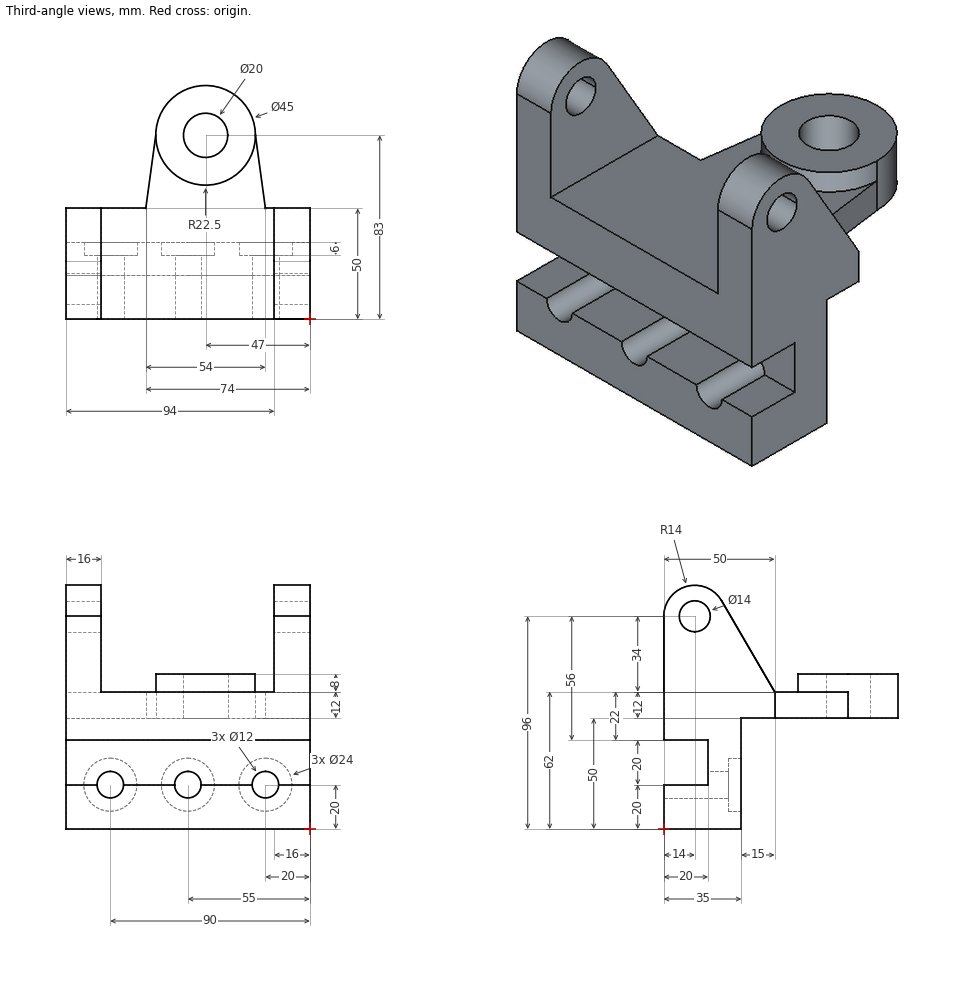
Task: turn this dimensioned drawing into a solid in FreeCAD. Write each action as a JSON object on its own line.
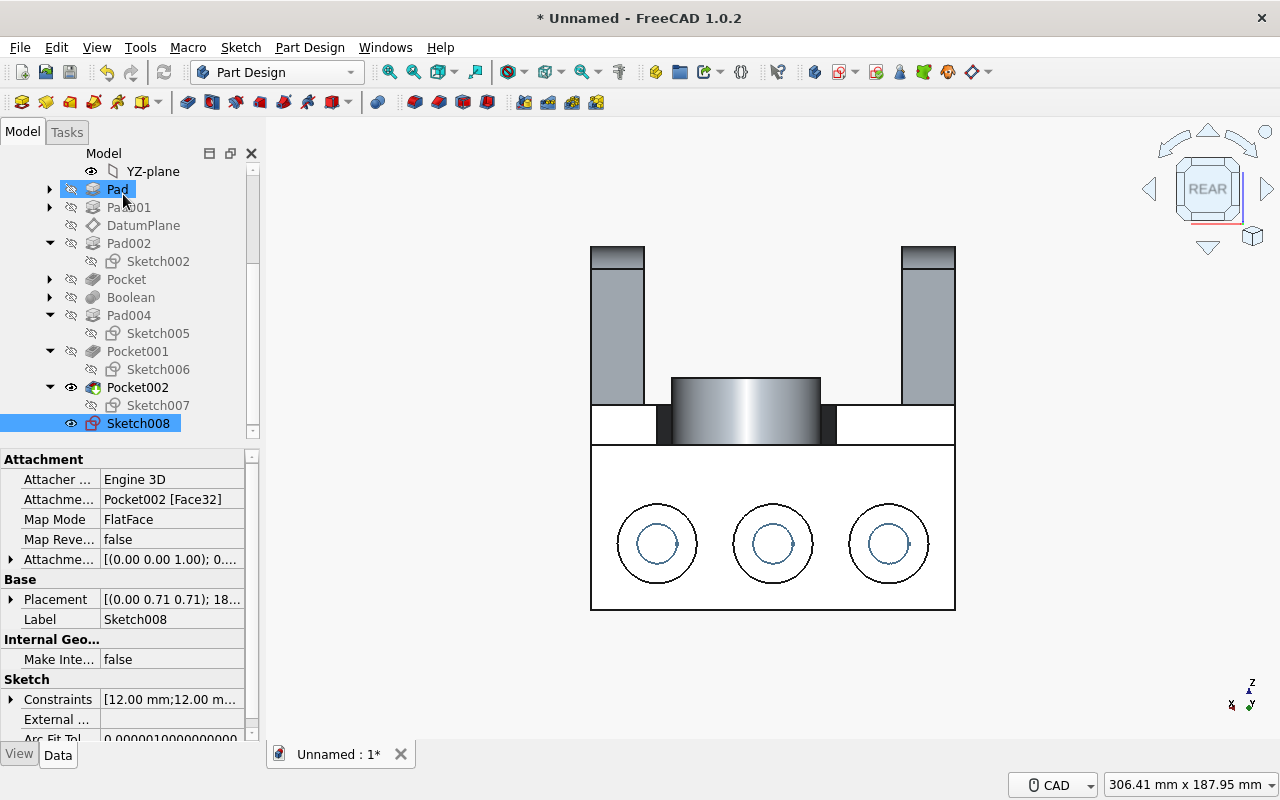
{"action": "left_click", "coordinate": [188, 102]}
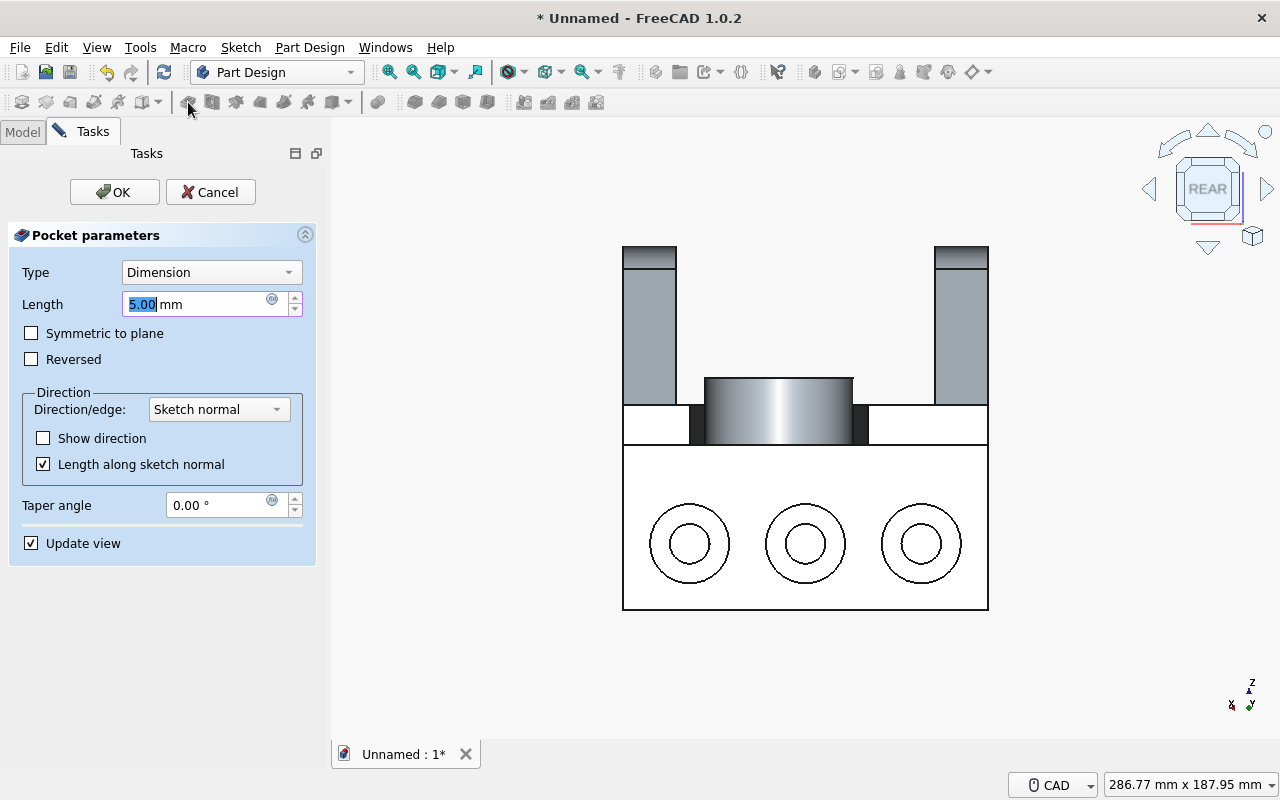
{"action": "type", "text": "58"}
{"action": "key", "text": "Tab"}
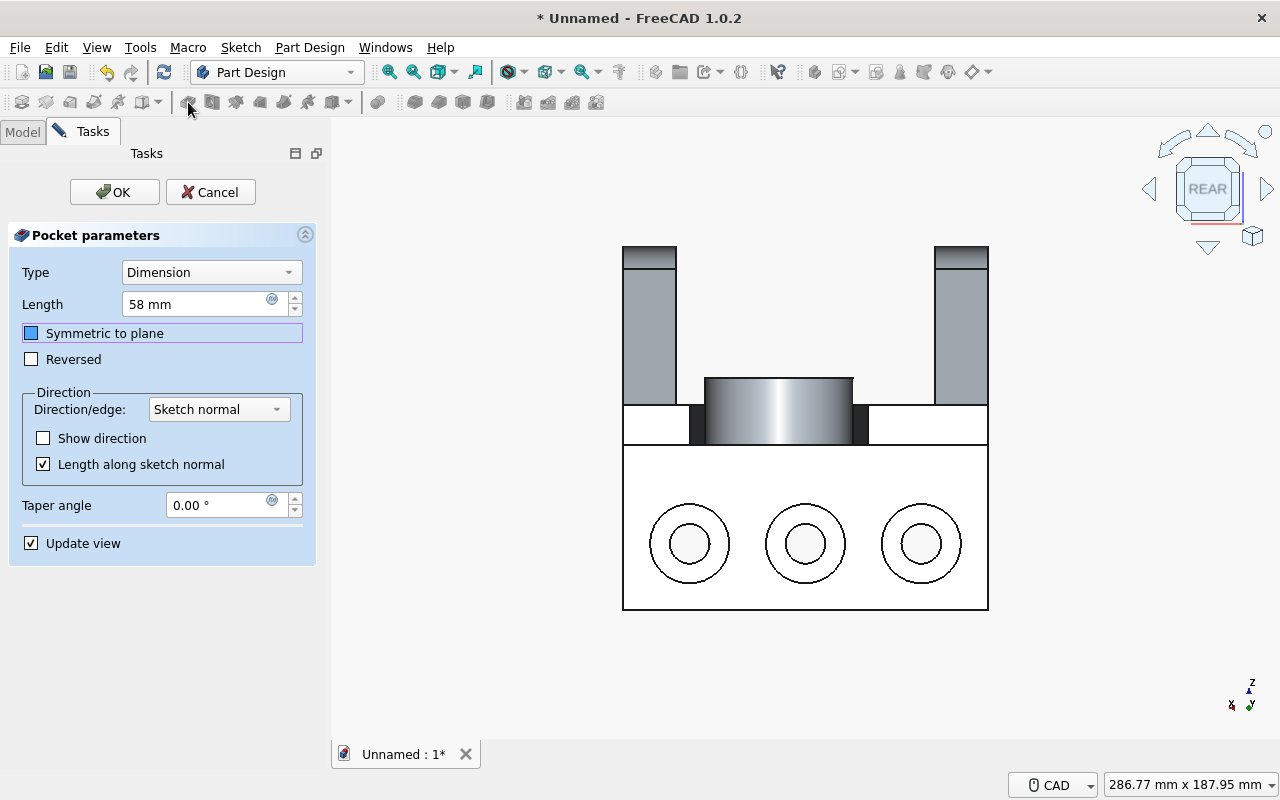
{"action": "left_click", "coordinate": [115, 192]}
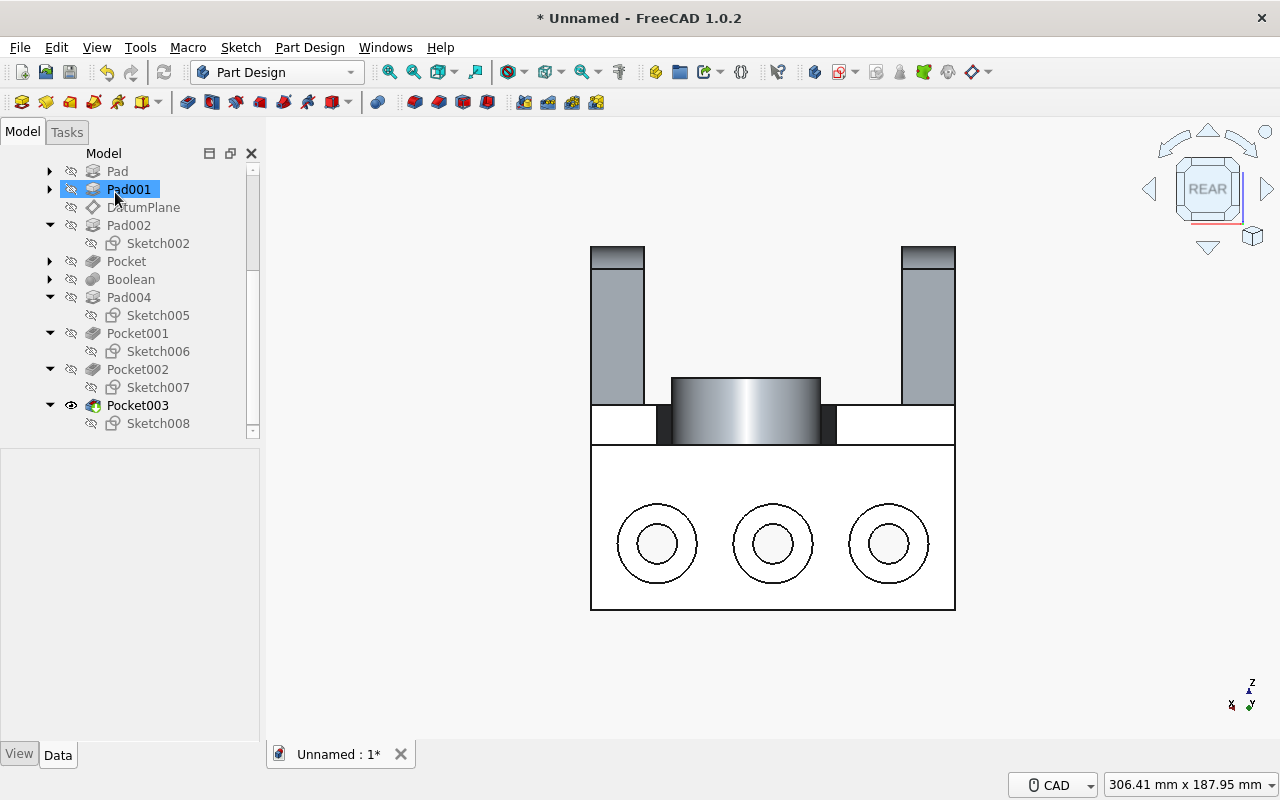
{"action": "key", "text": "0"}